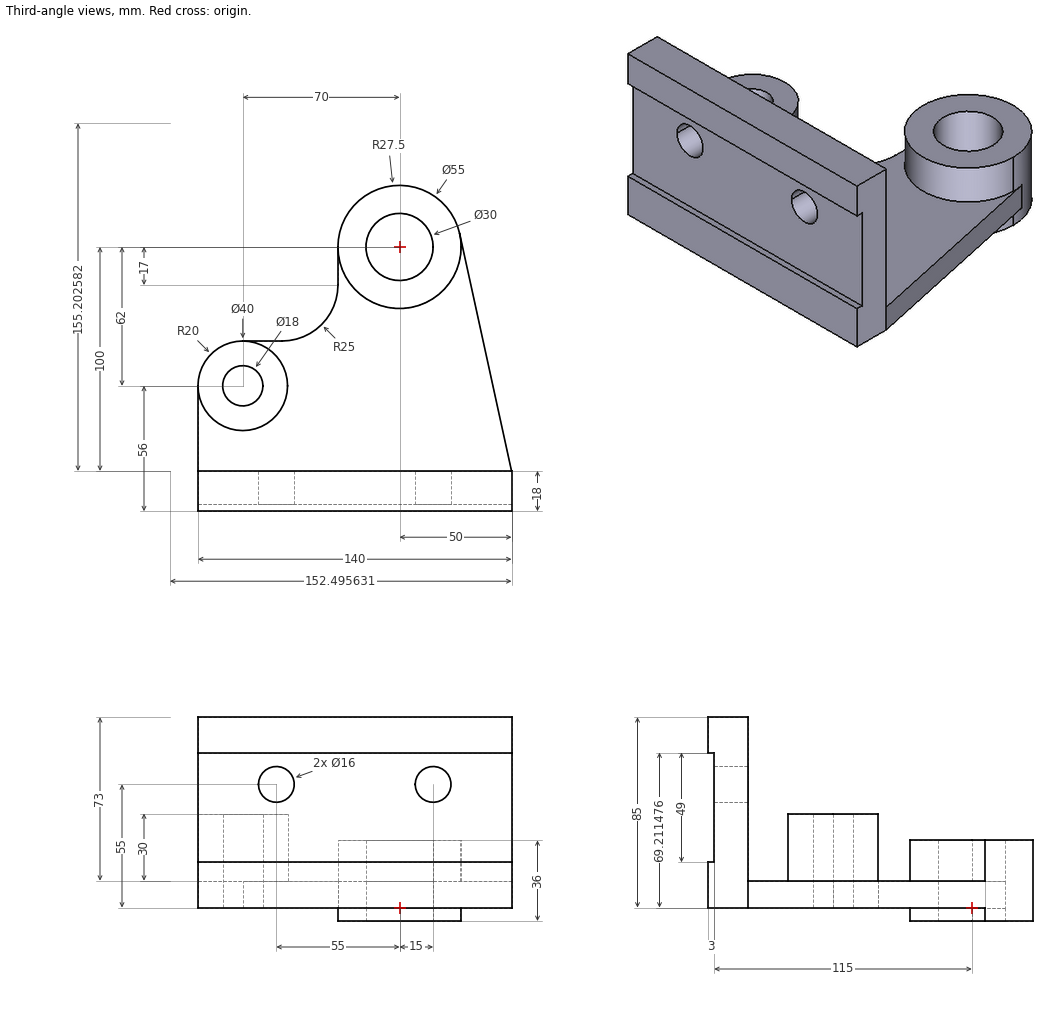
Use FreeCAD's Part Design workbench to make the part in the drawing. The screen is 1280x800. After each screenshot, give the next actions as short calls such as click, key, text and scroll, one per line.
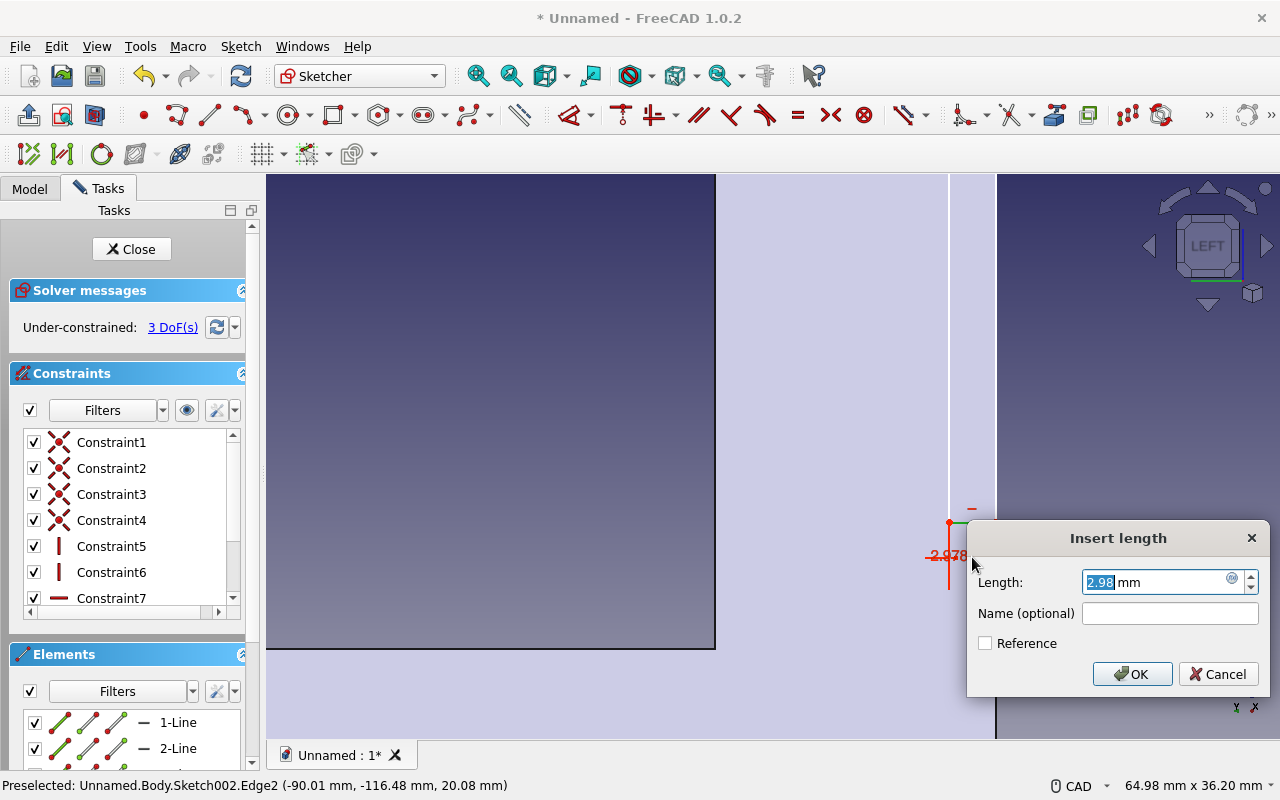
text(3)
key(Return)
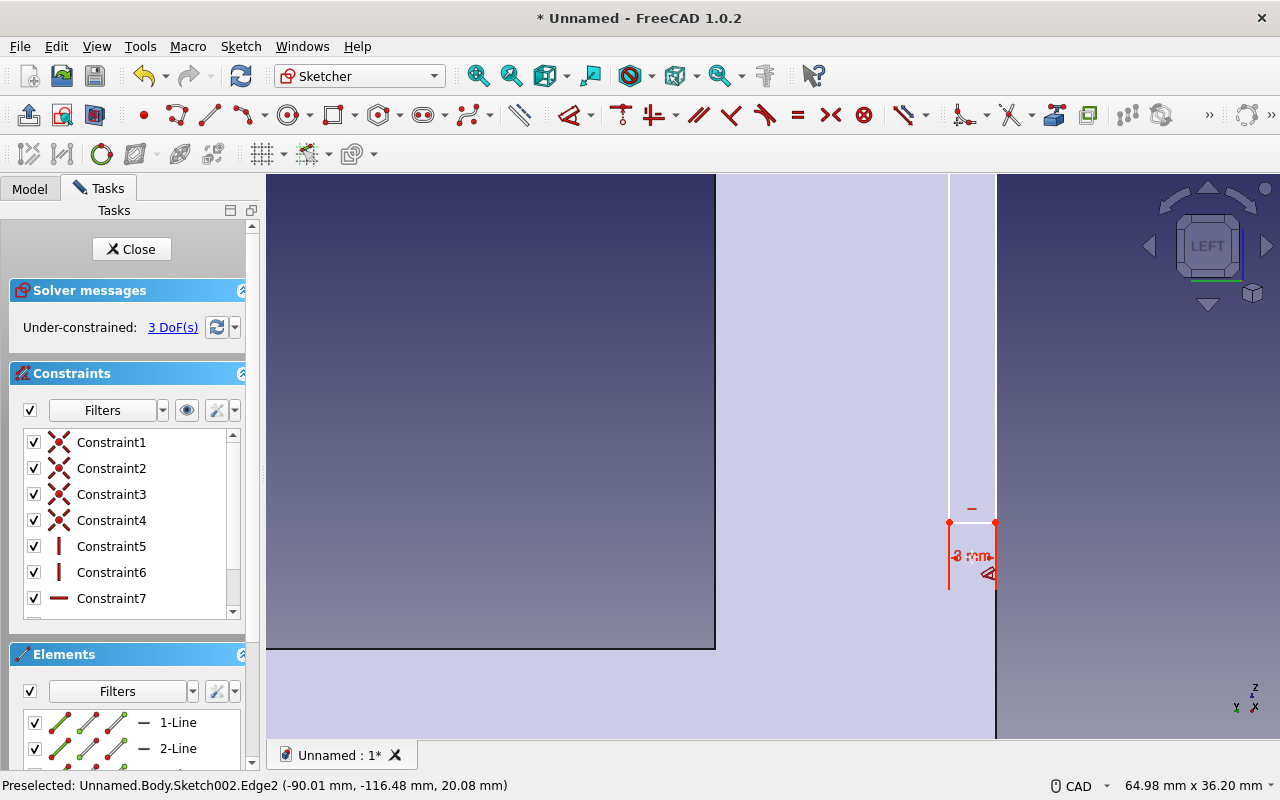
click(949, 293)
click(915, 362)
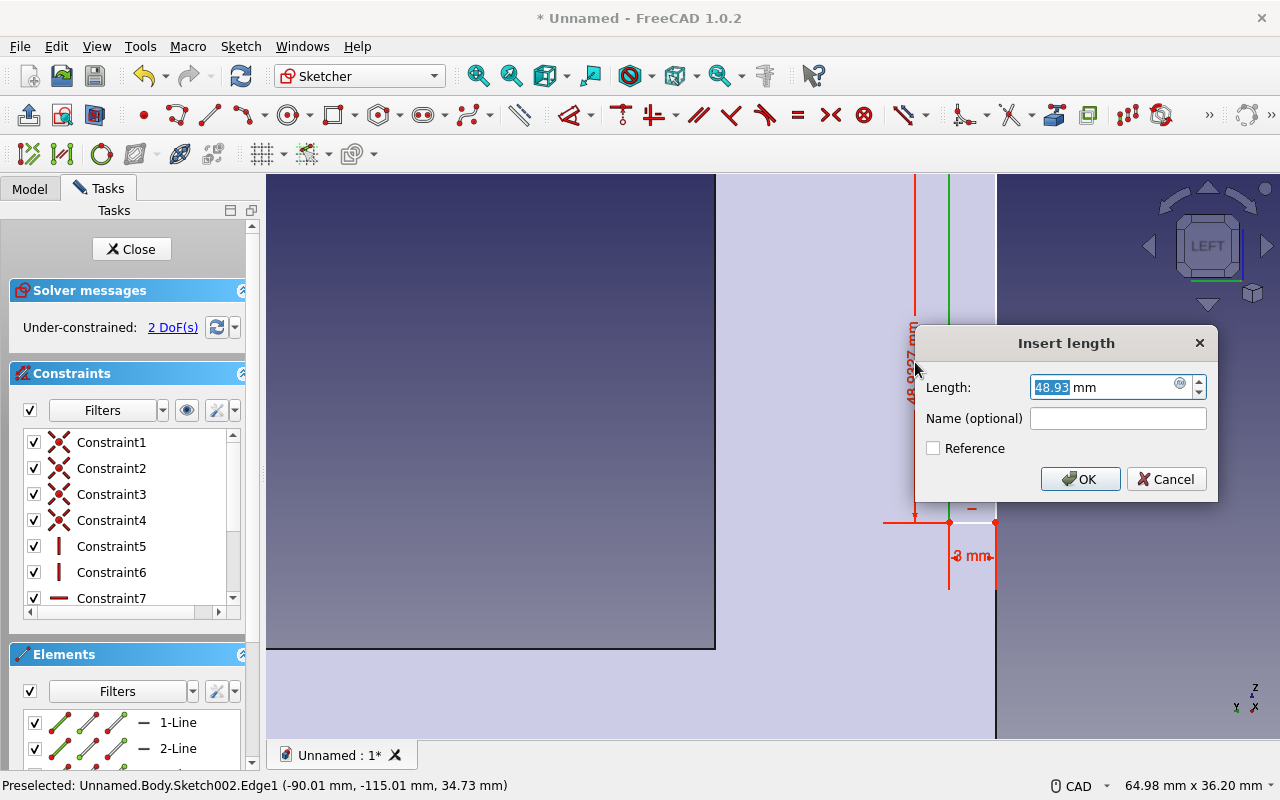
text(49)
key(Return)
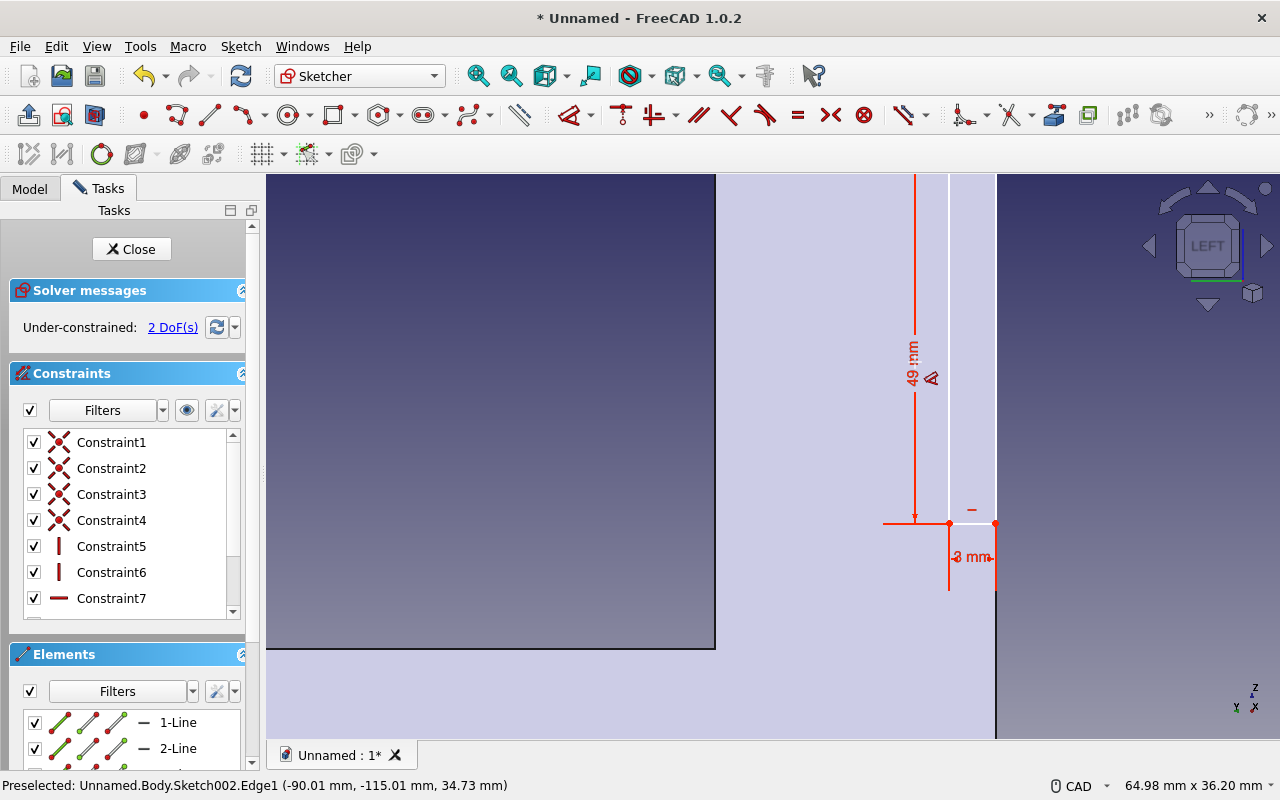
scroll(976, 526, down, 6)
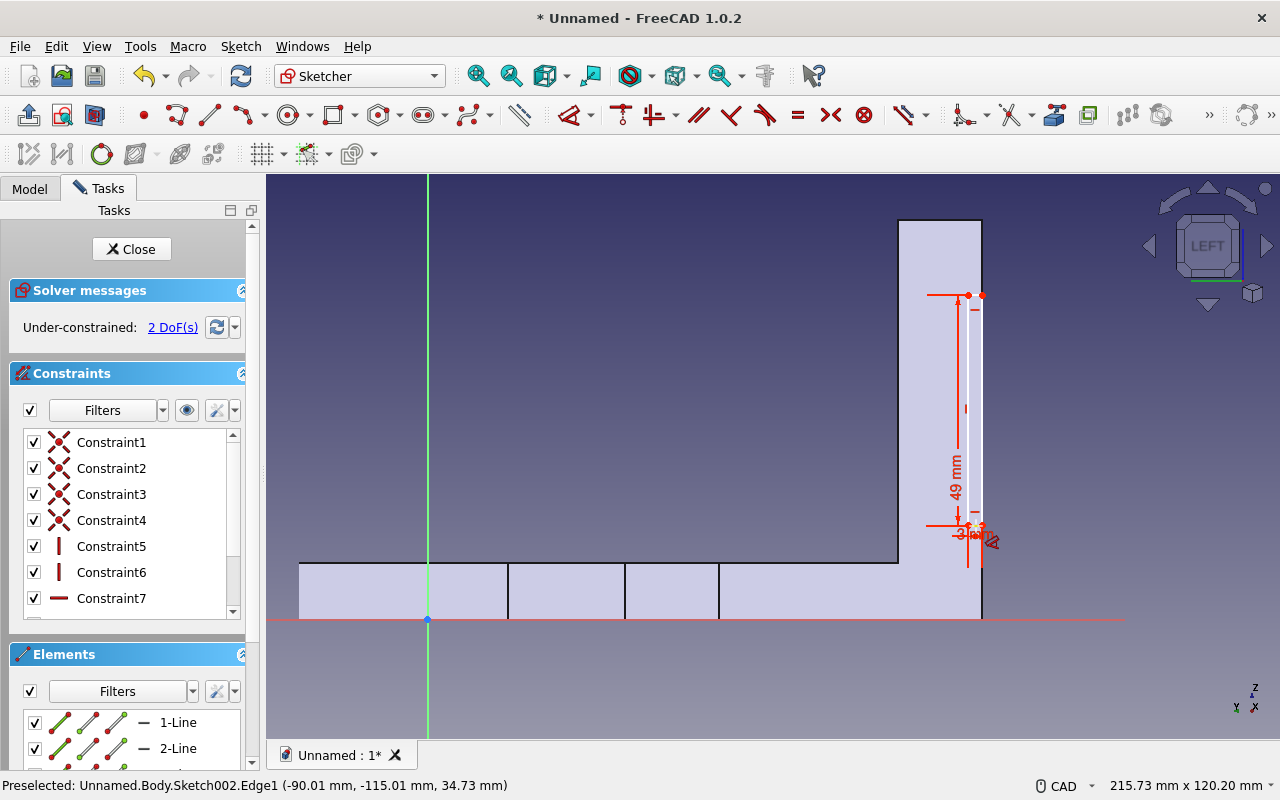
click(968, 295)
click(698, 654)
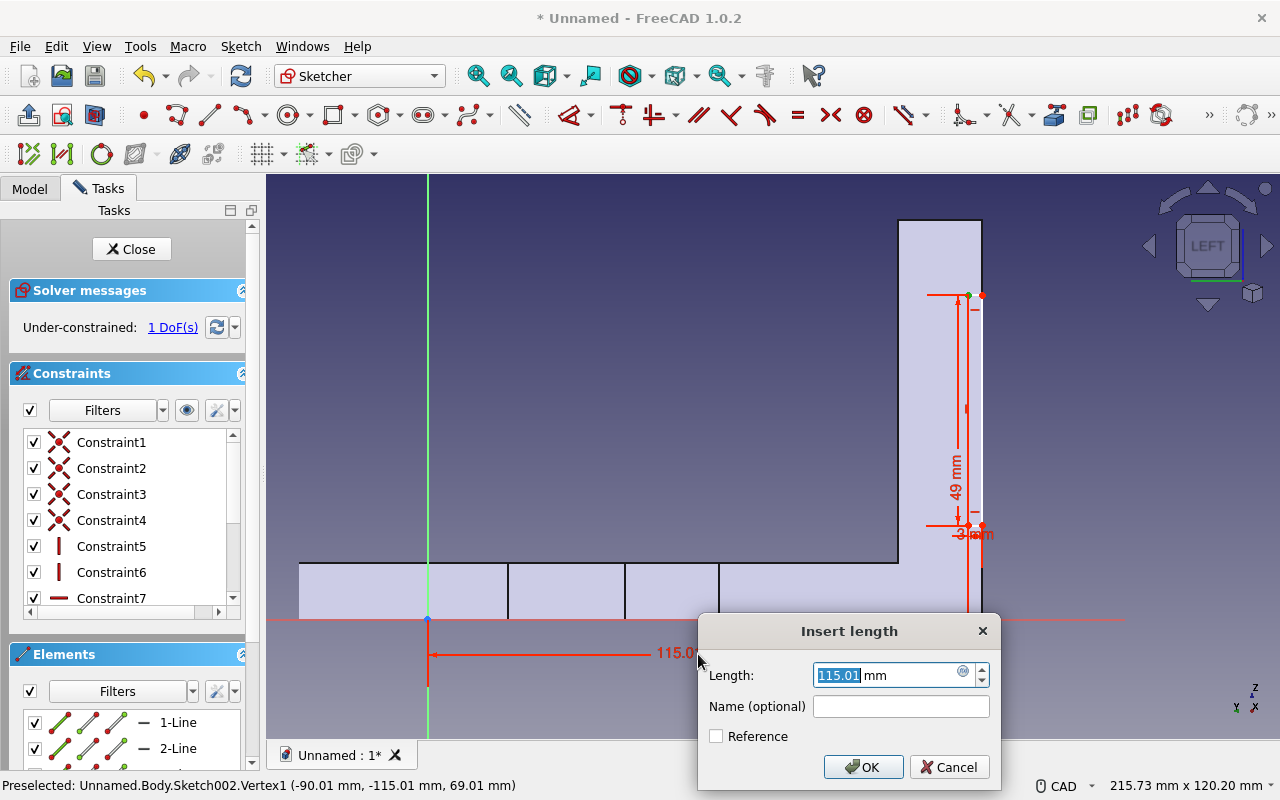
text(115)
key(Return)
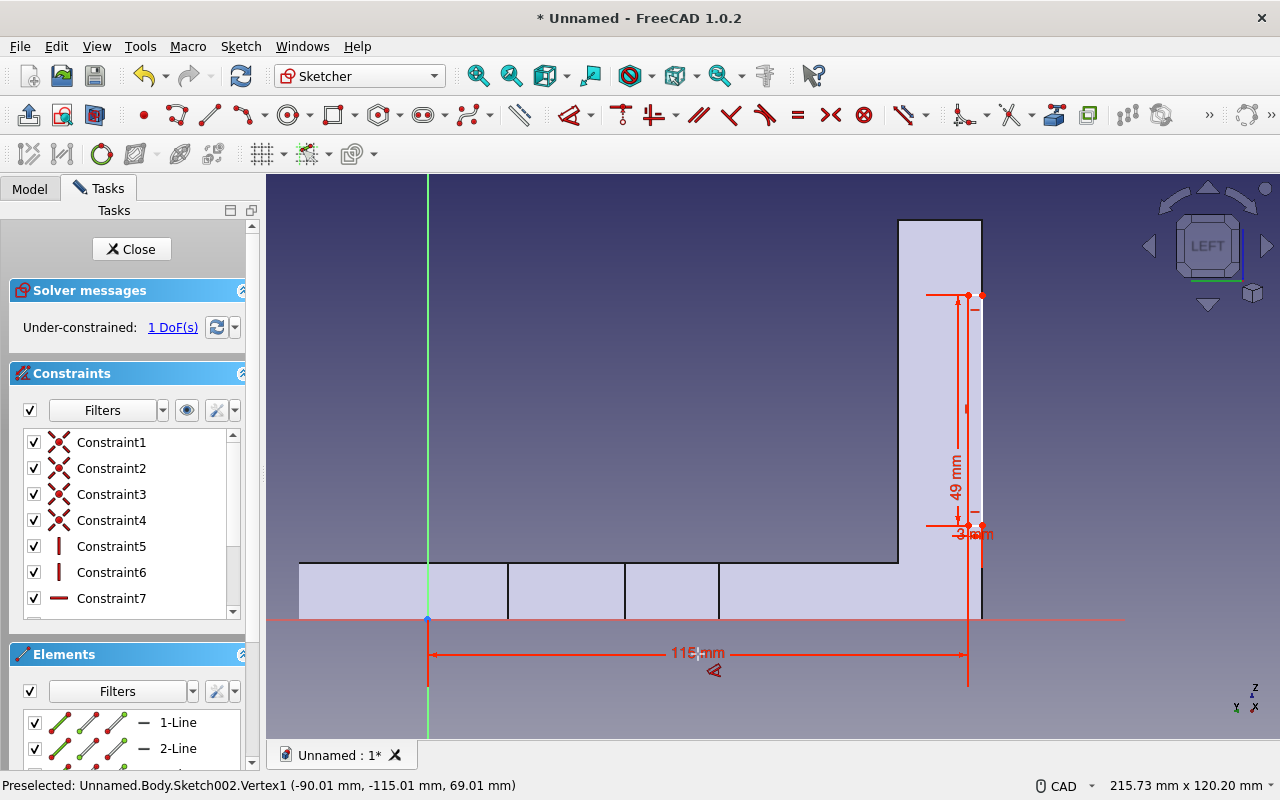
click(968, 295)
click(394, 458)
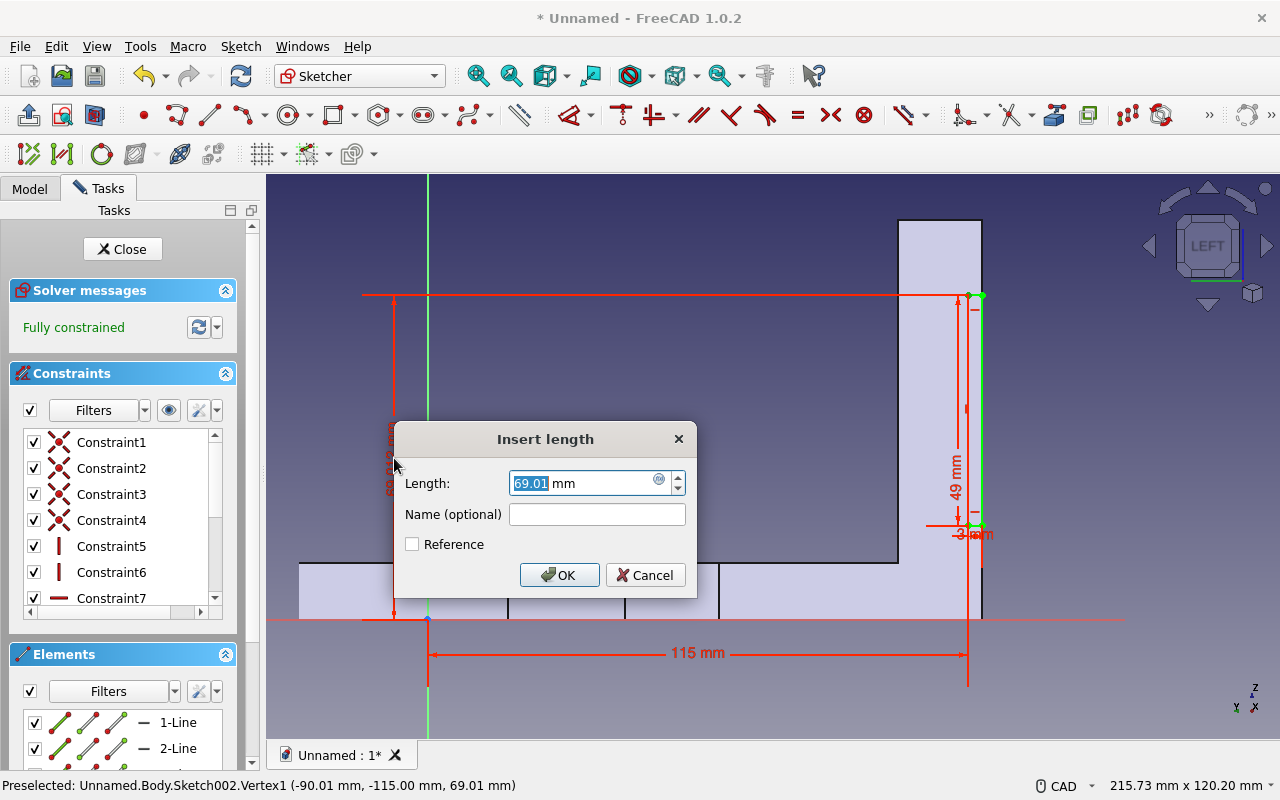
text(69.211476)
key(Return)
key(Escape)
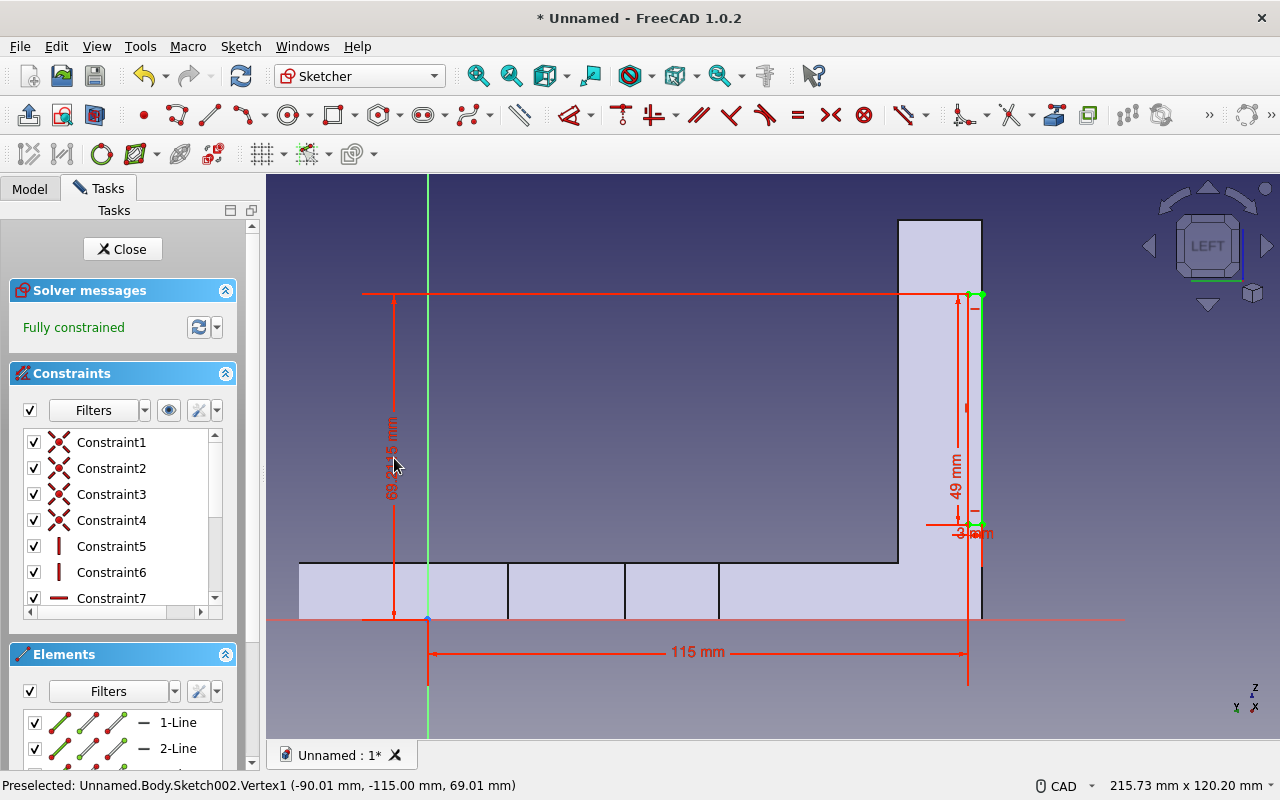
click(123, 249)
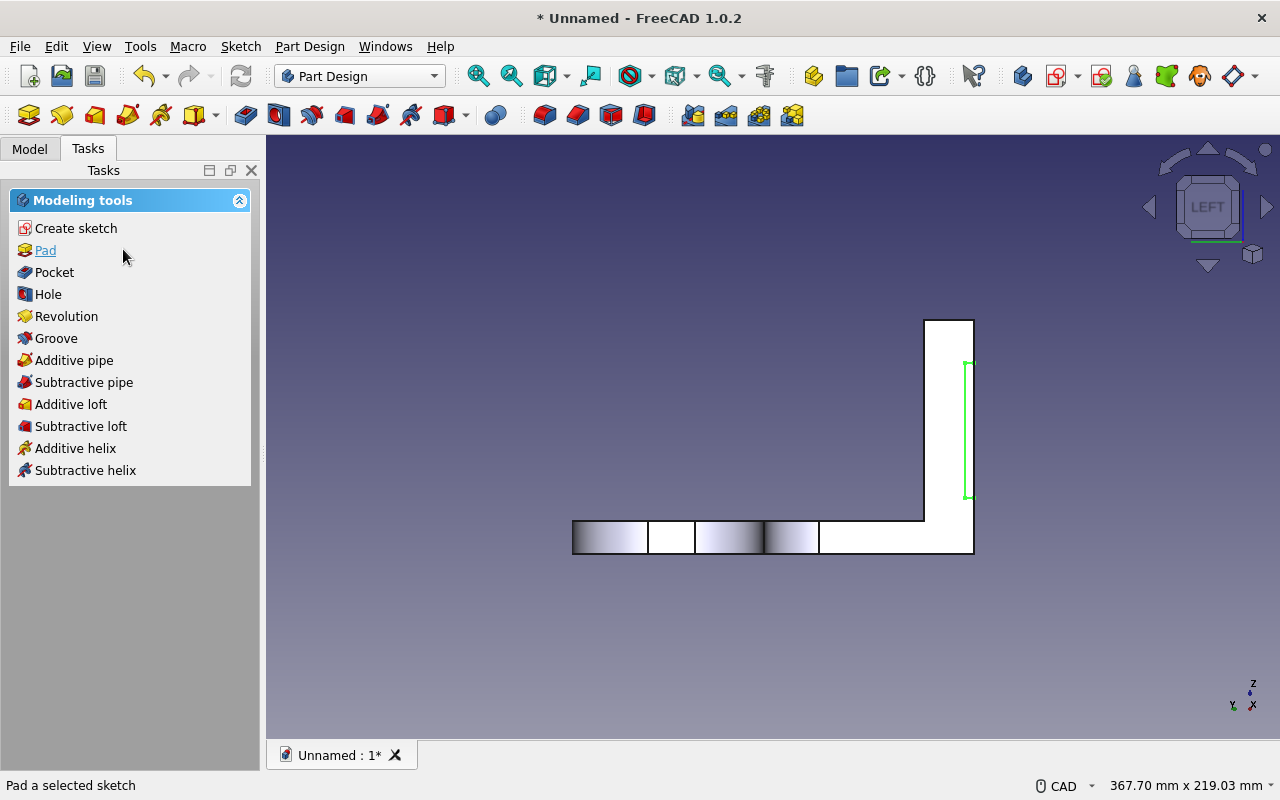
click(246, 116)